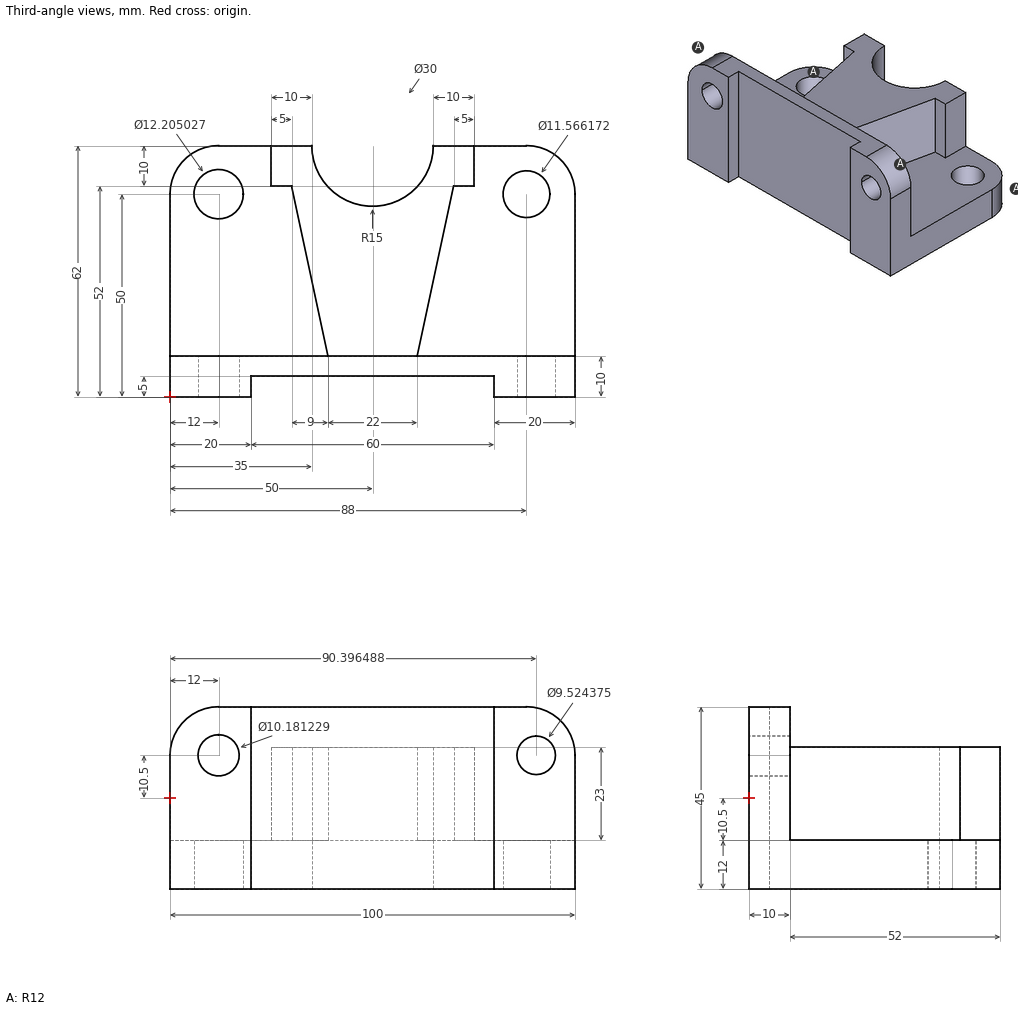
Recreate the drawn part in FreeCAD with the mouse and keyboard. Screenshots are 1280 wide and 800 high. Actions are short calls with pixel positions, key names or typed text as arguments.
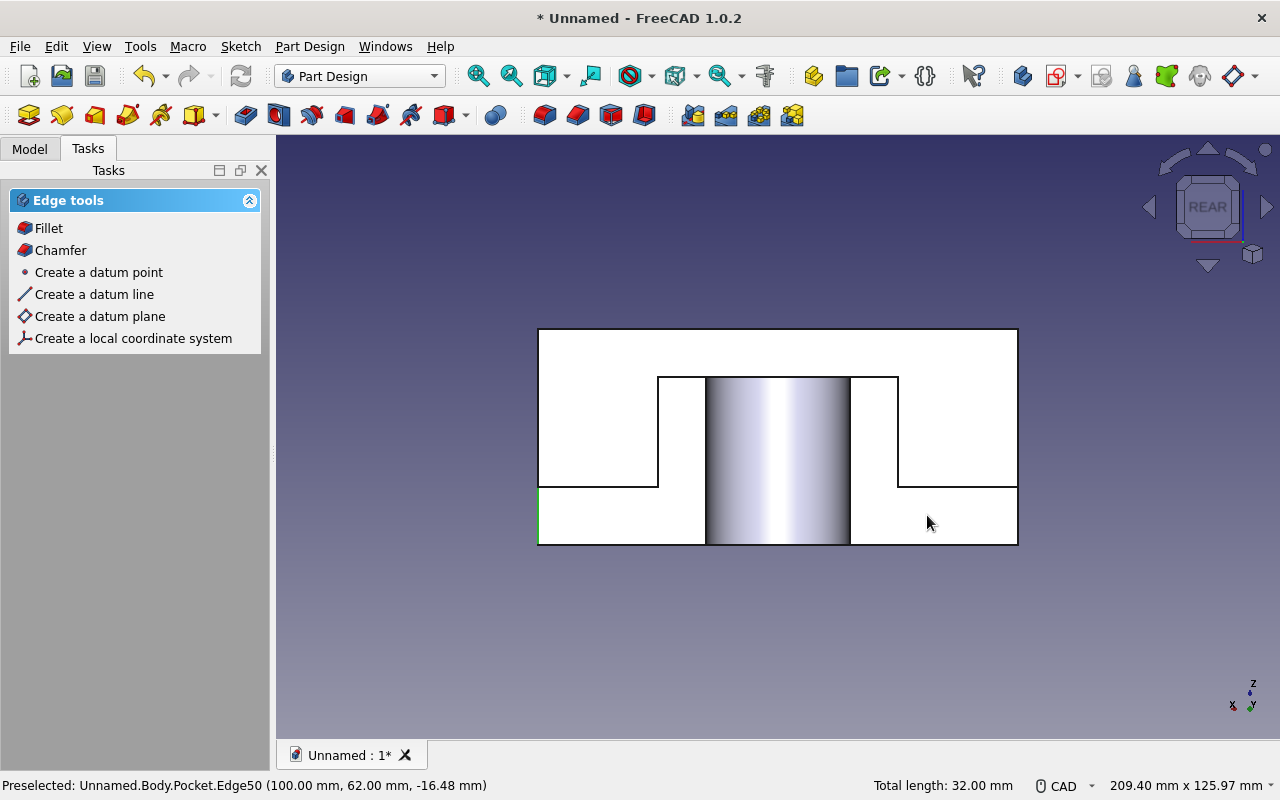
click(1018, 515, ctrl)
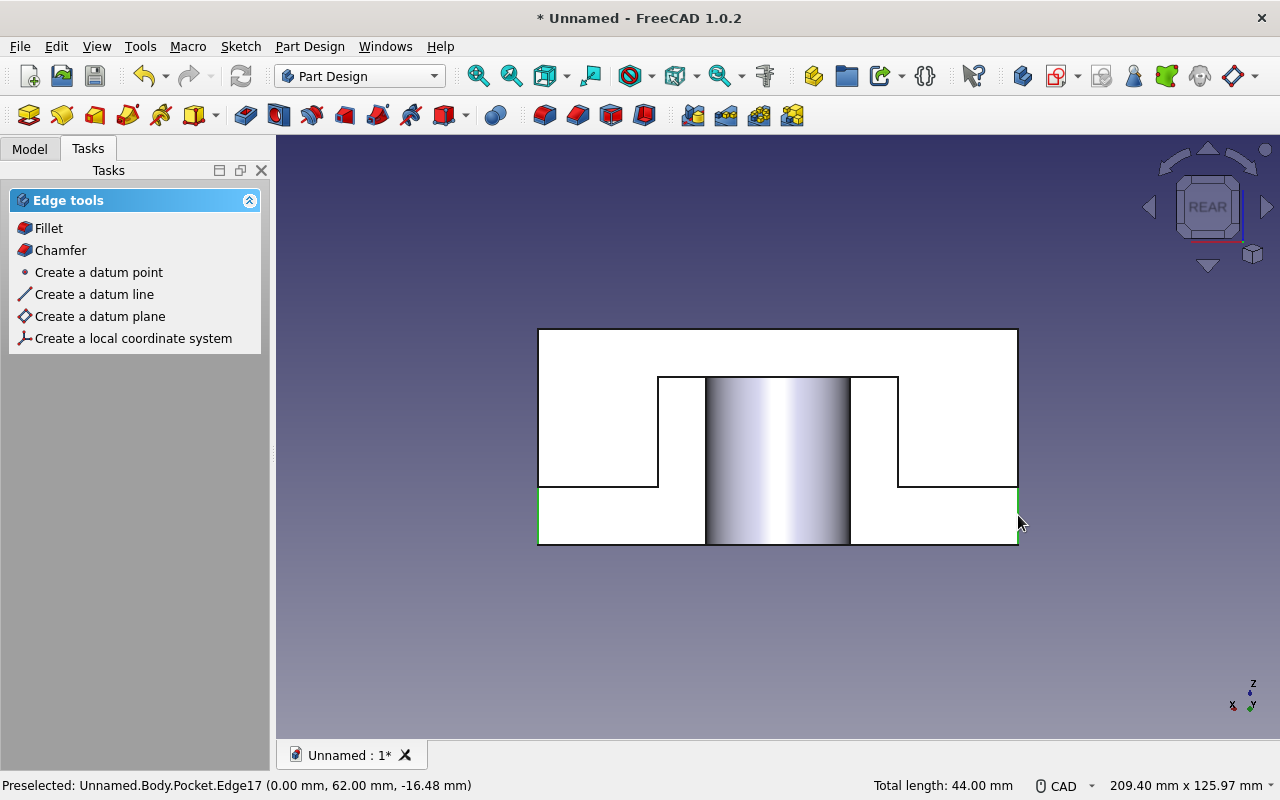
click(545, 116)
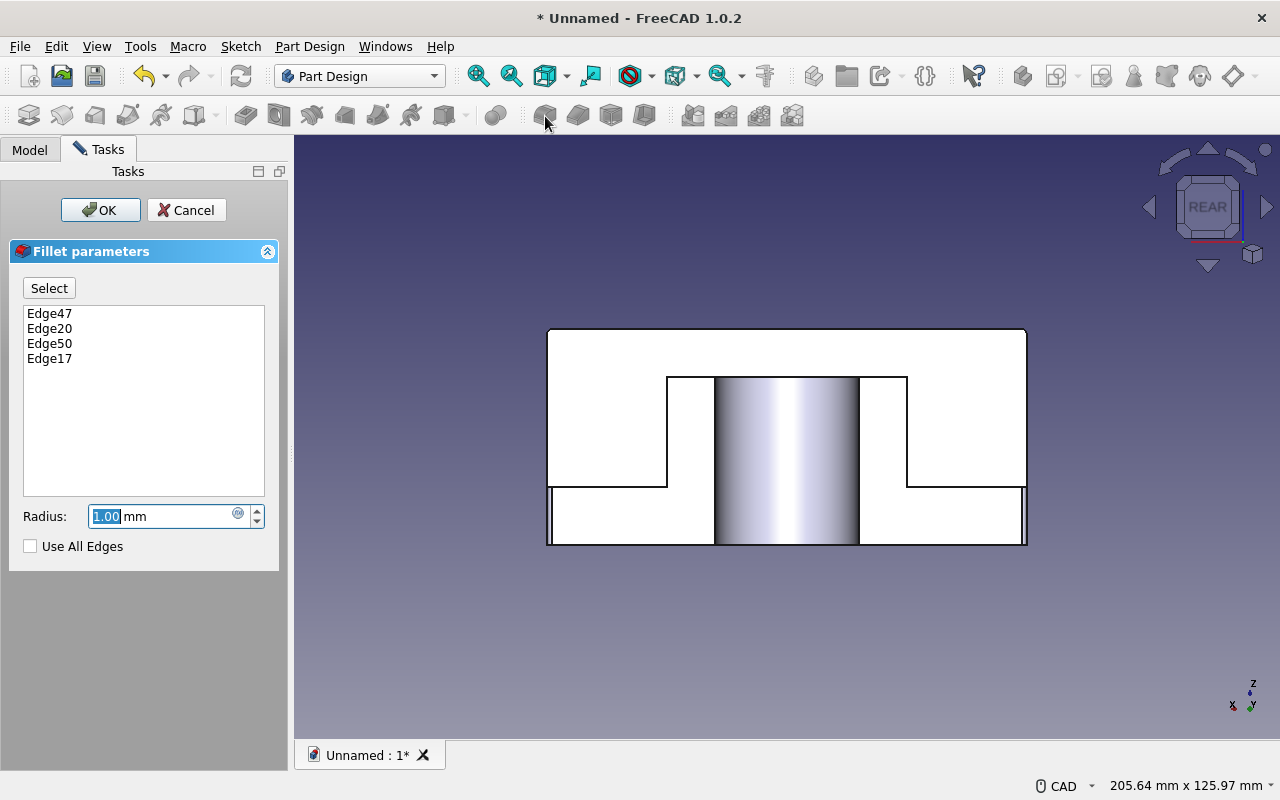
text(12)
key(Tab)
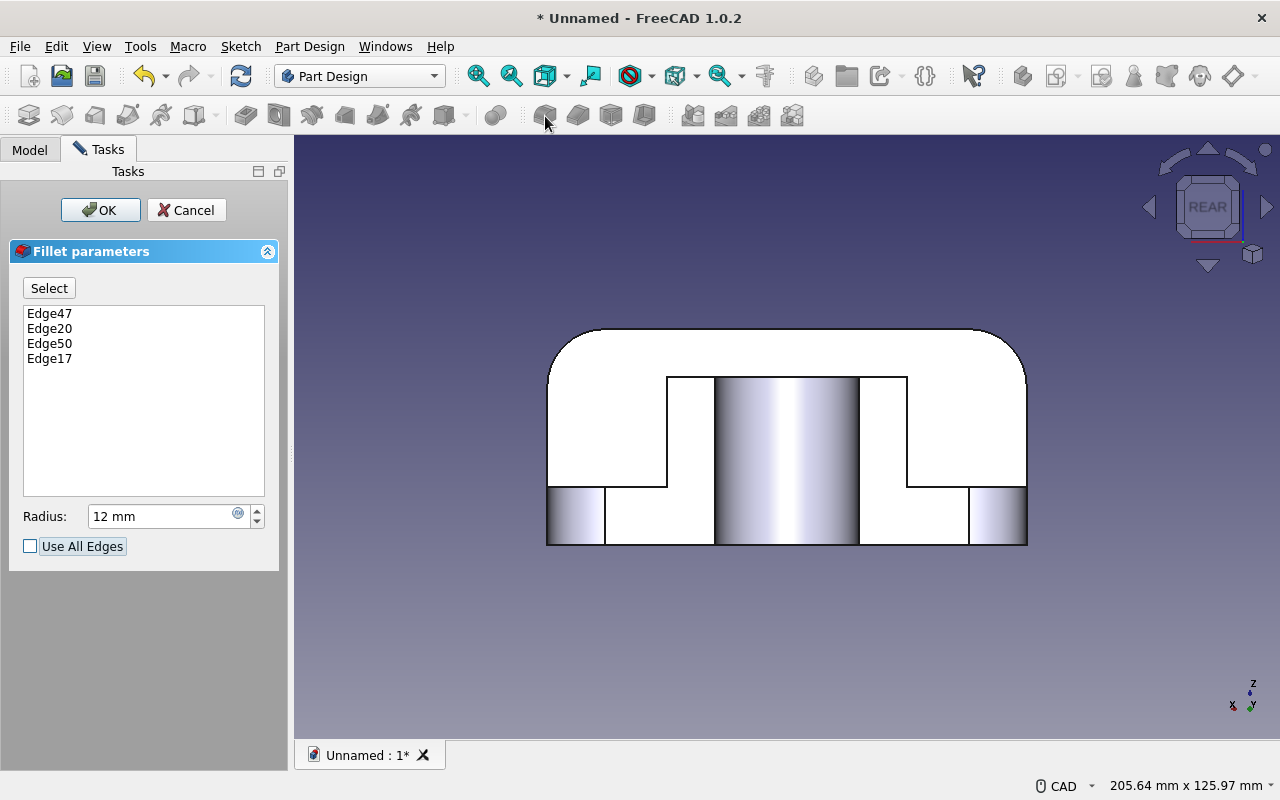
click(101, 210)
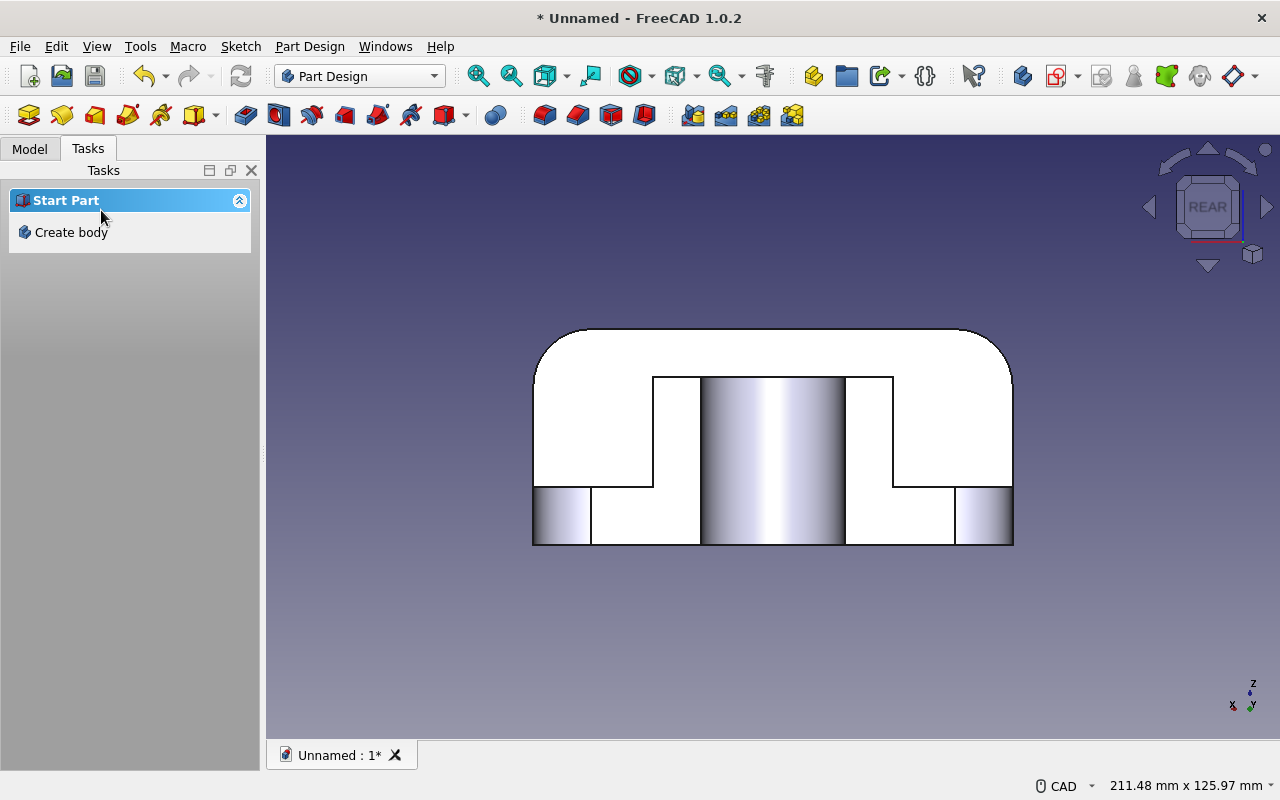
click(636, 407)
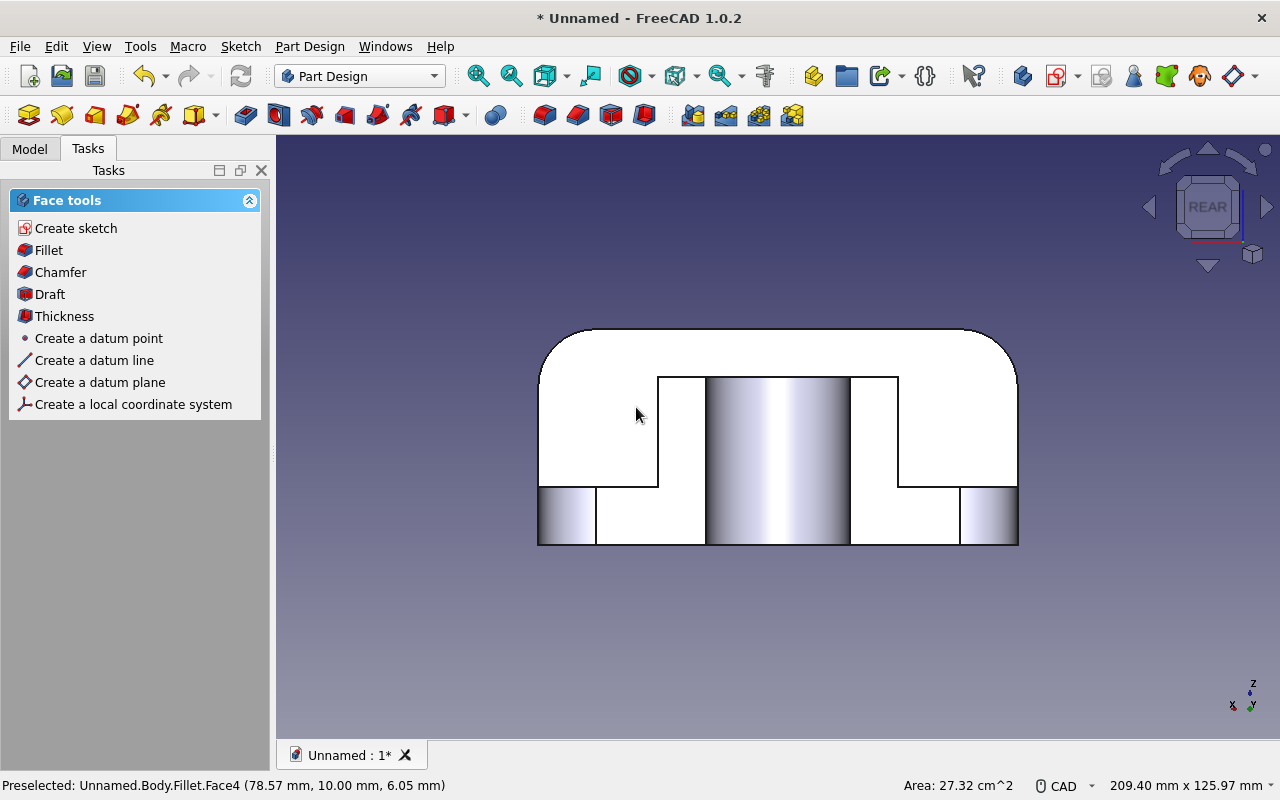
click(1056, 76)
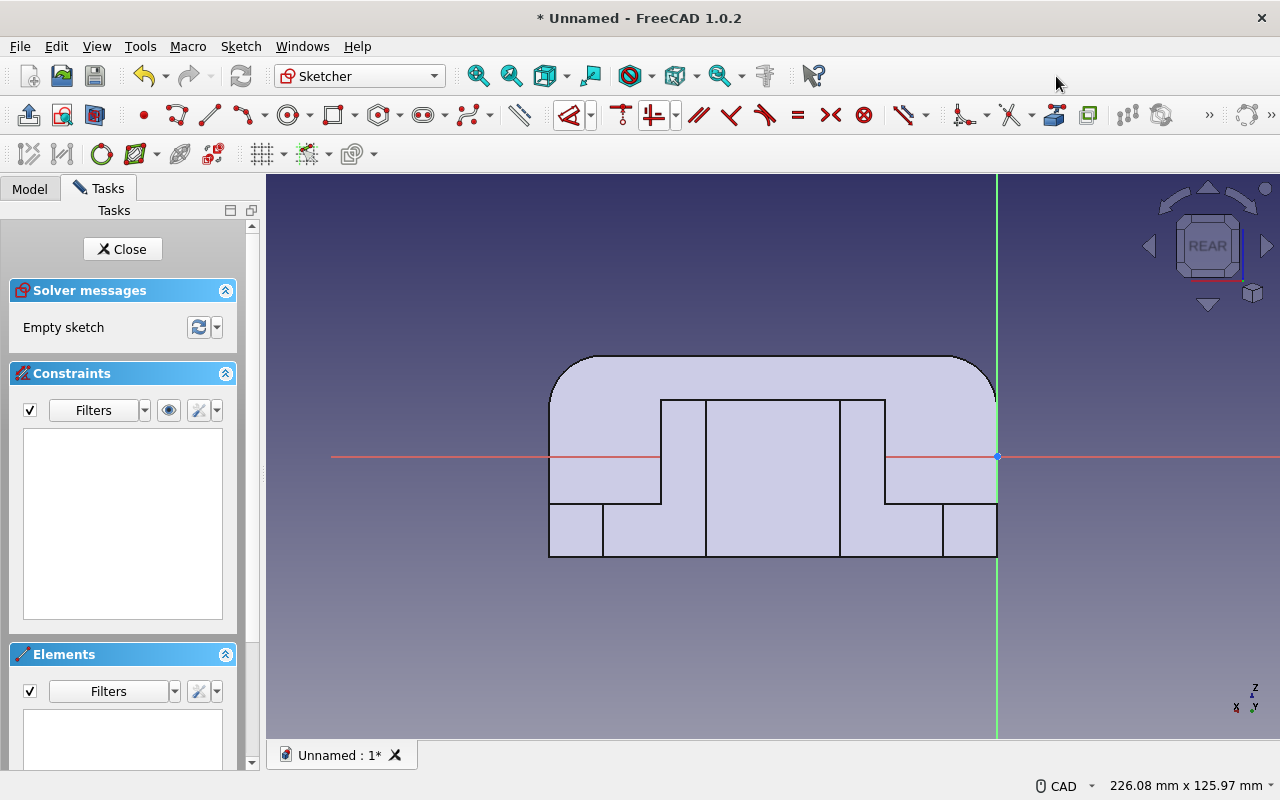
scroll(945, 350, up, 2)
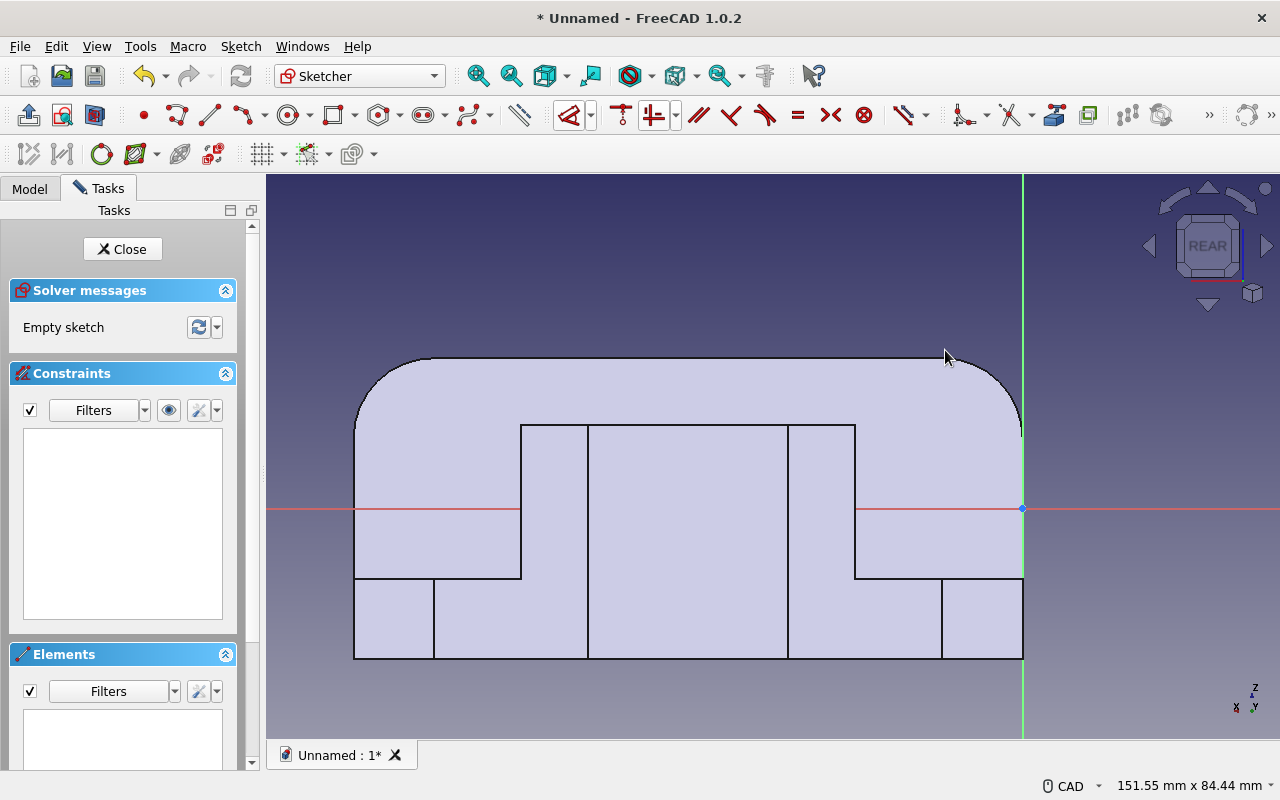
key(g)
key(c)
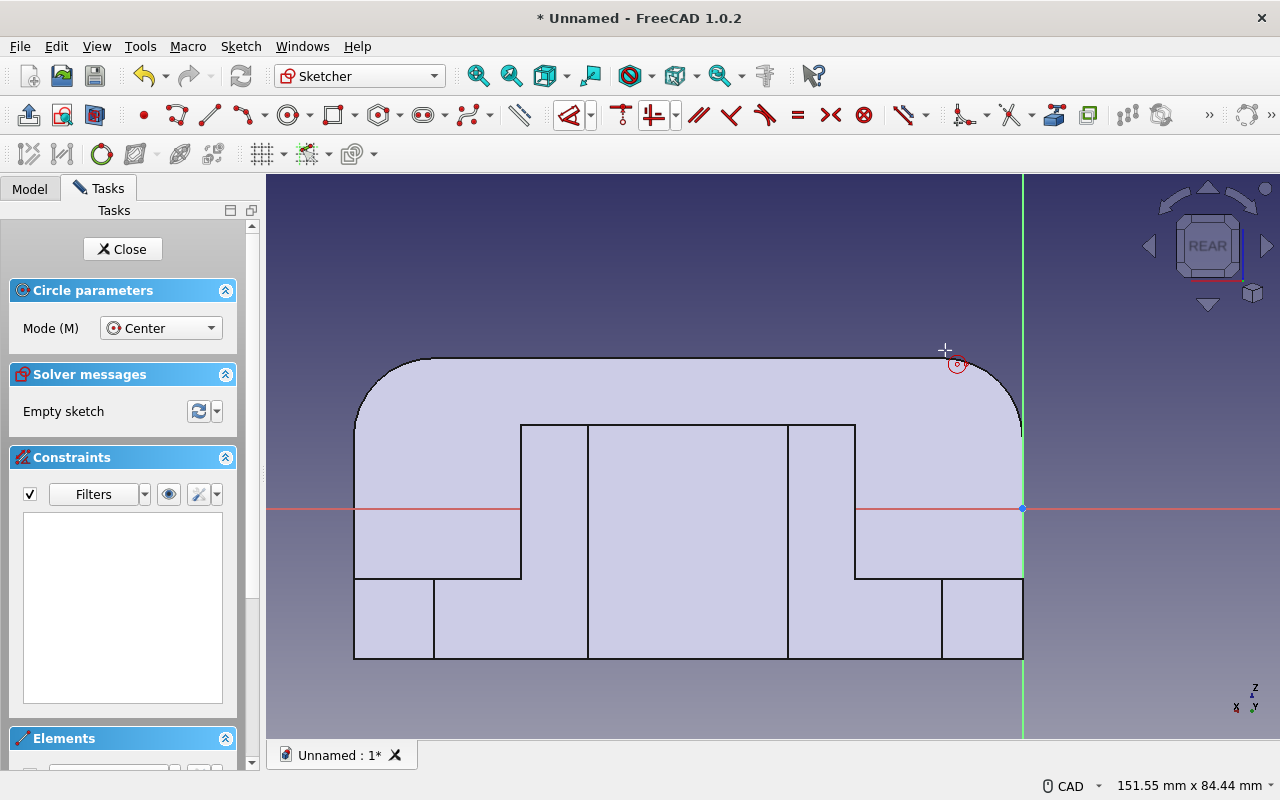
click(942, 438)
click(966, 414)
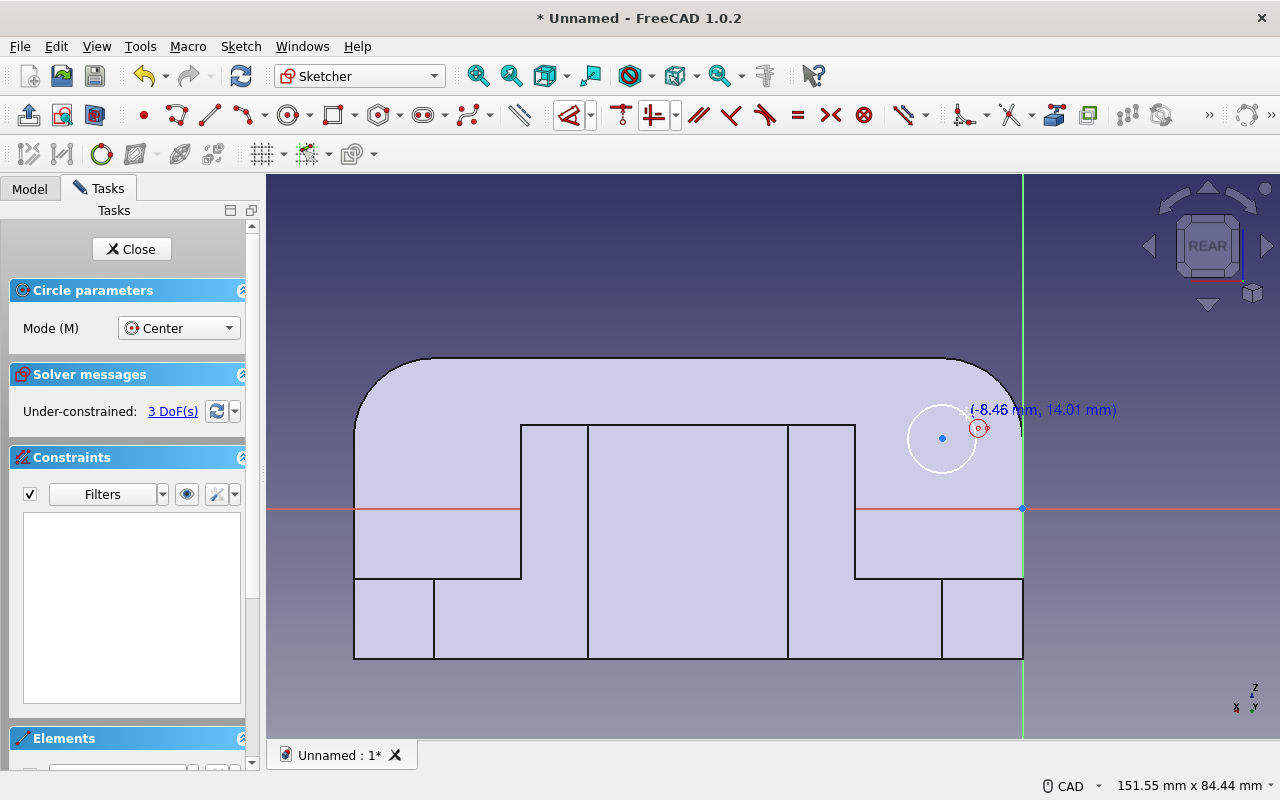
click(418, 438)
click(440, 416)
key(Escape)